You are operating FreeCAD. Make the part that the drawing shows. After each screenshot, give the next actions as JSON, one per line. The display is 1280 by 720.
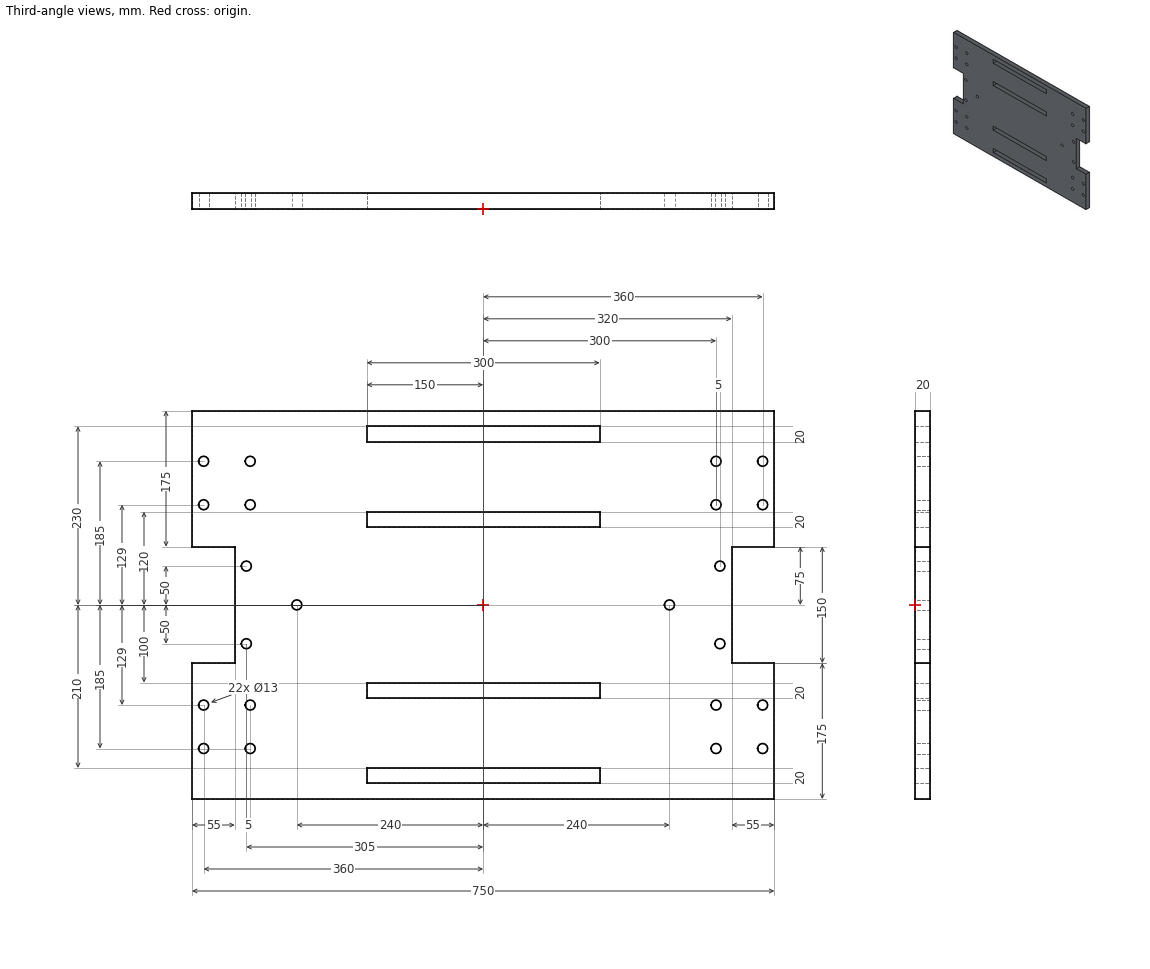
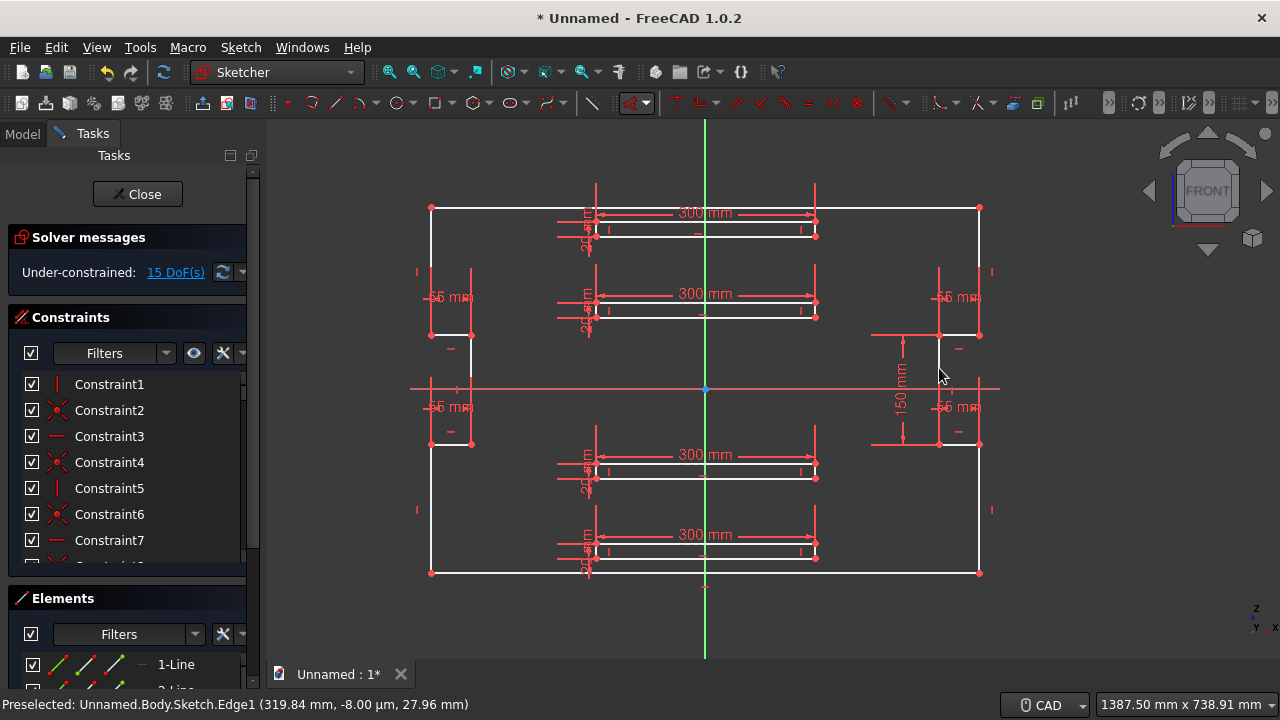
{"action": "left_click", "coordinate": [979, 483]}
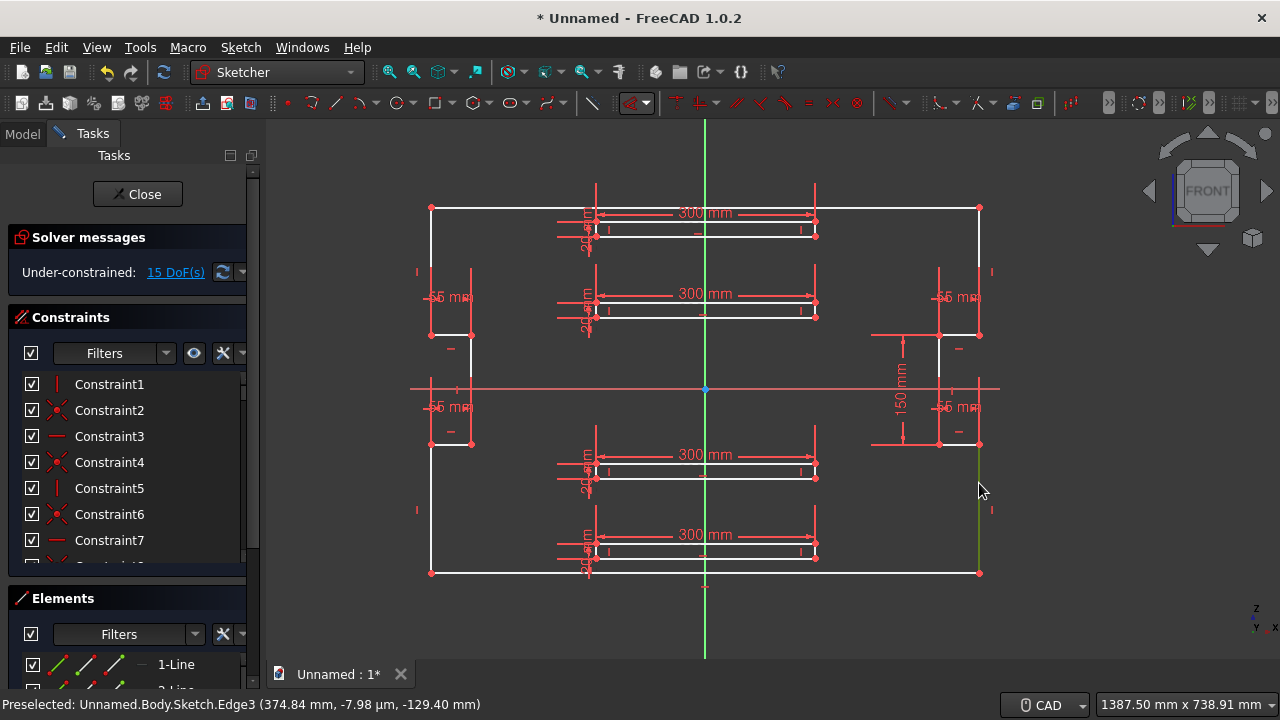
{"action": "left_click", "coordinate": [648, 104]}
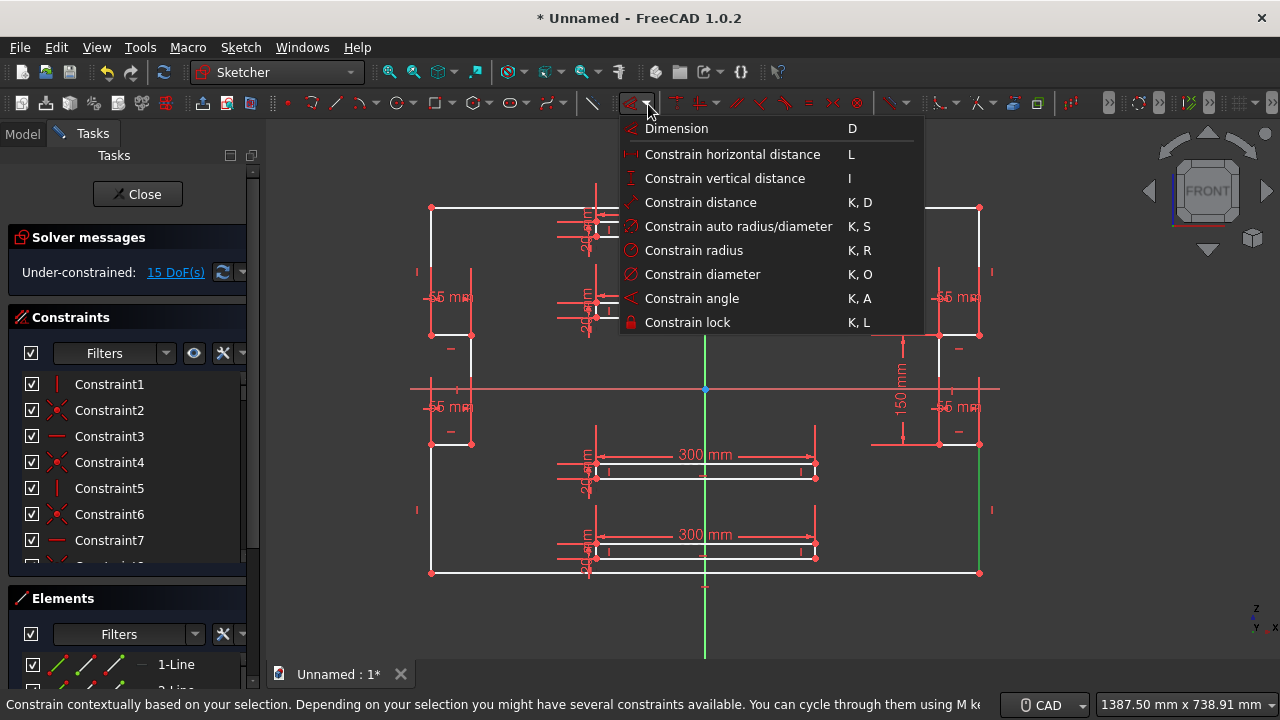
{"action": "left_click", "coordinate": [772, 178]}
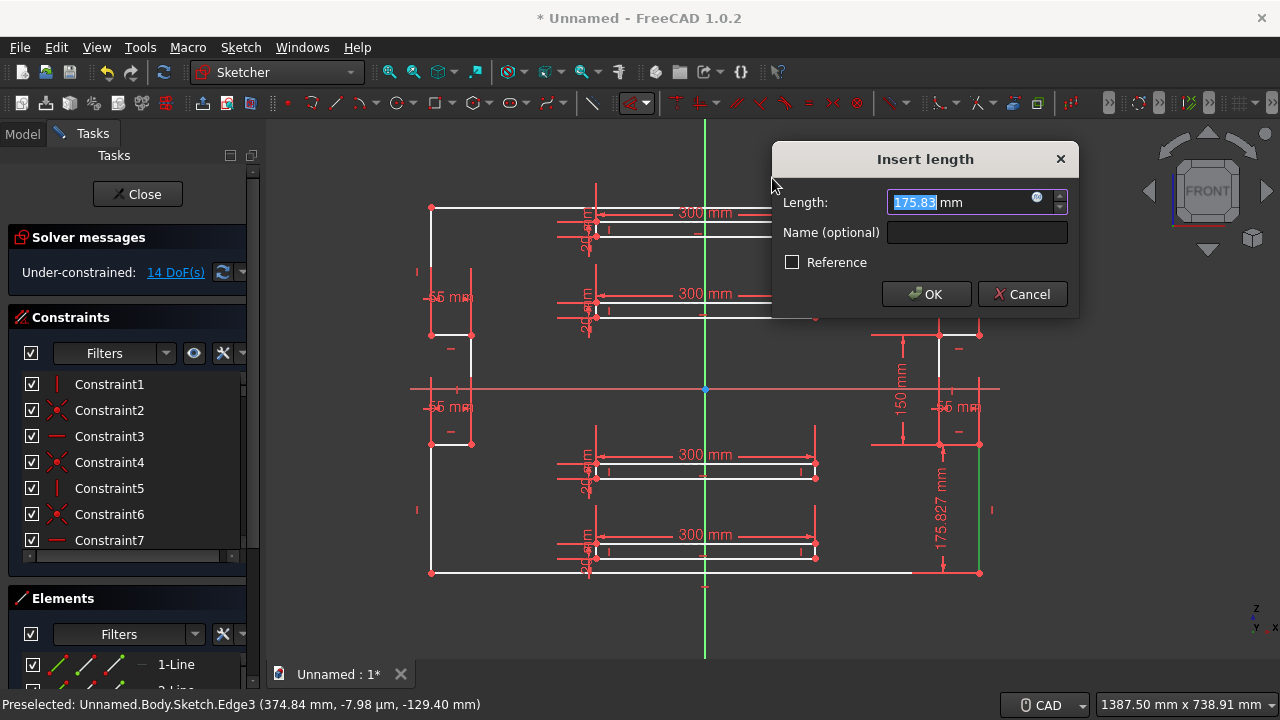
{"action": "type", "text": "175"}
{"action": "key", "text": "Return"}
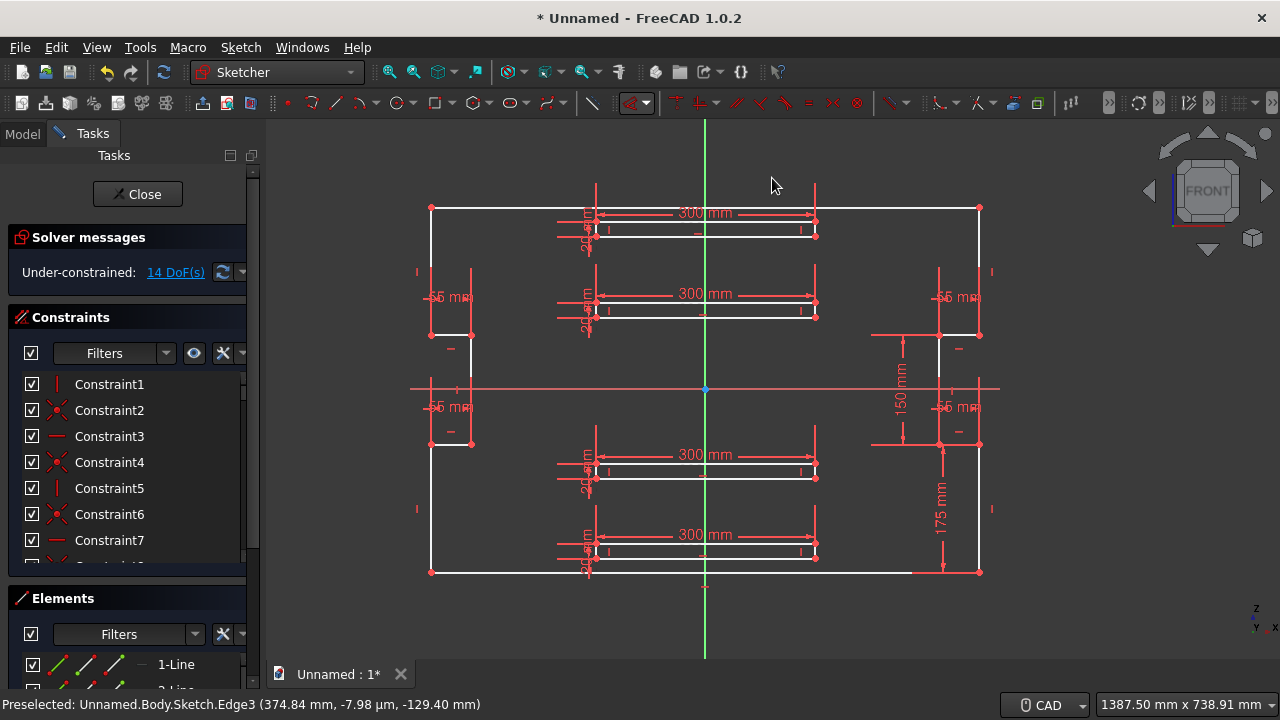
{"action": "left_click", "coordinate": [815, 573]}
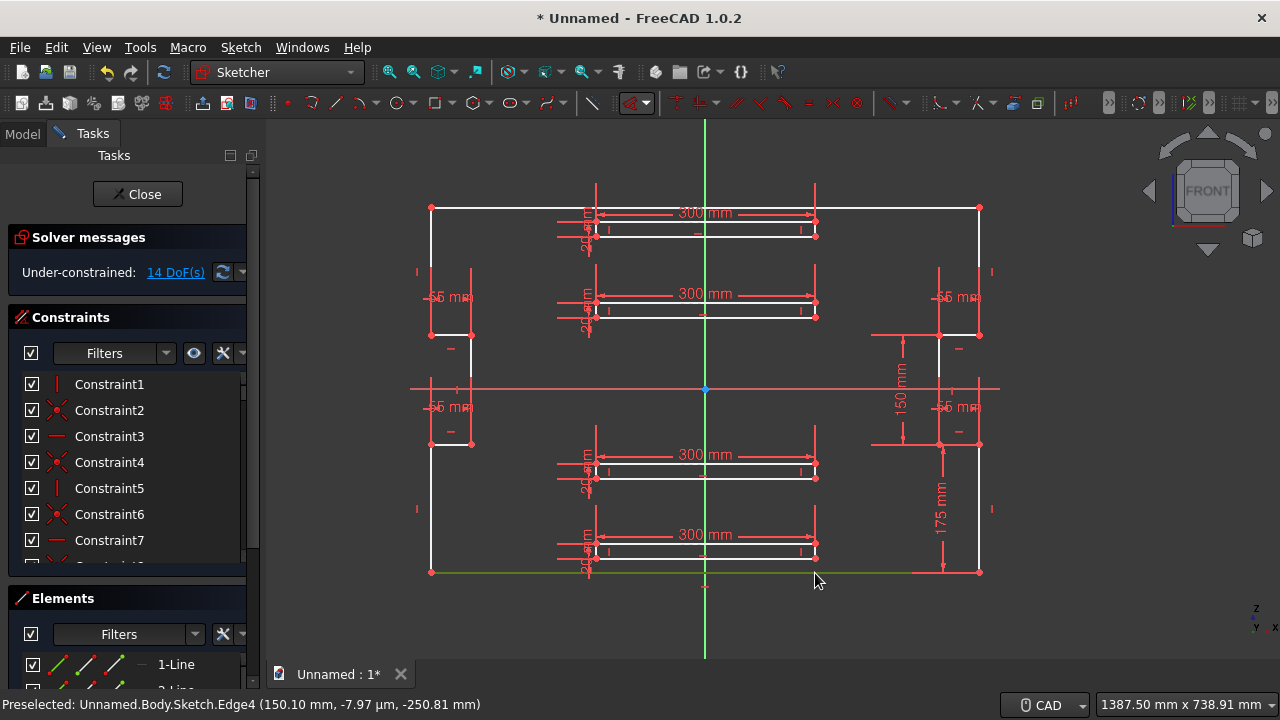
{"action": "left_click", "coordinate": [648, 104]}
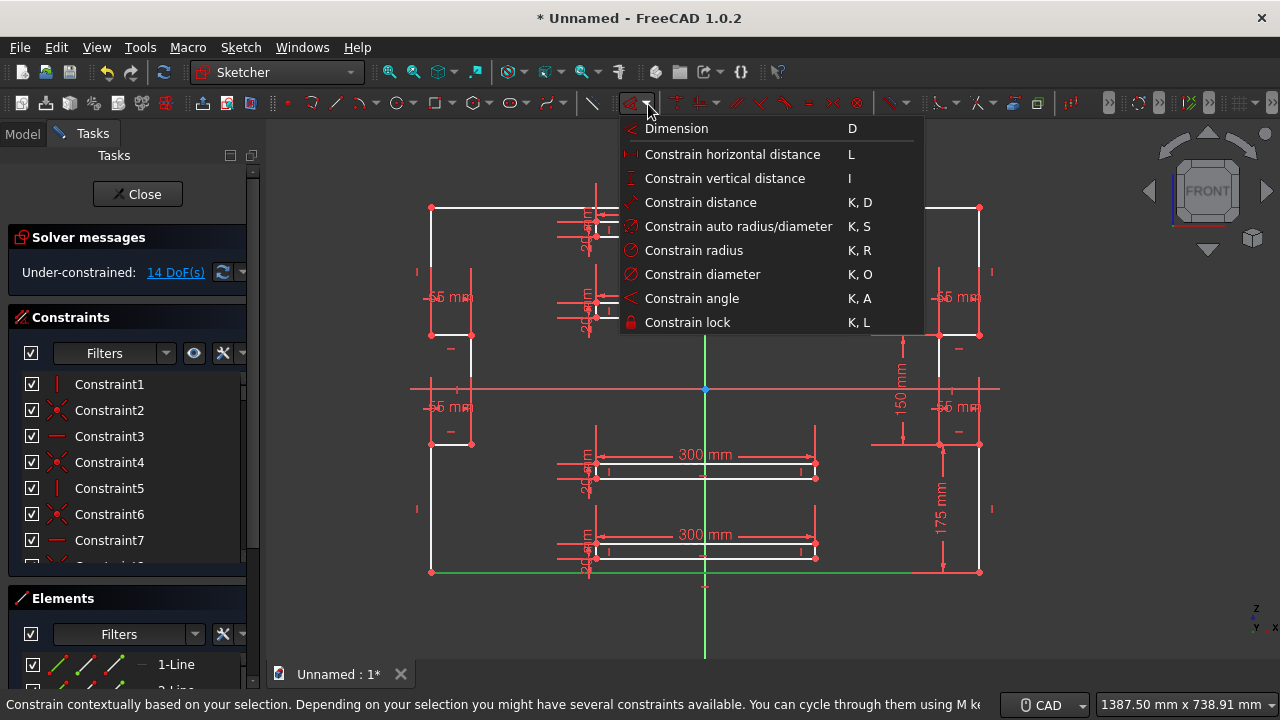
{"action": "left_click", "coordinate": [772, 154]}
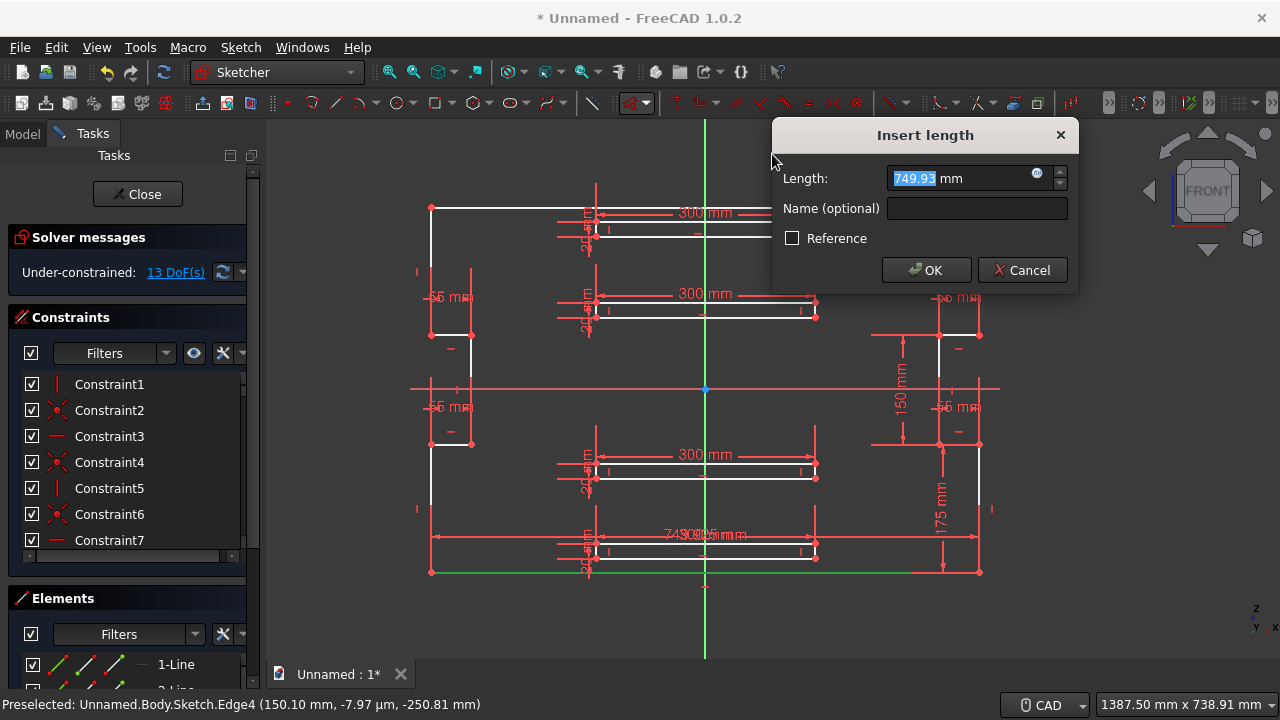
{"action": "type", "text": "750"}
{"action": "key", "text": "Return"}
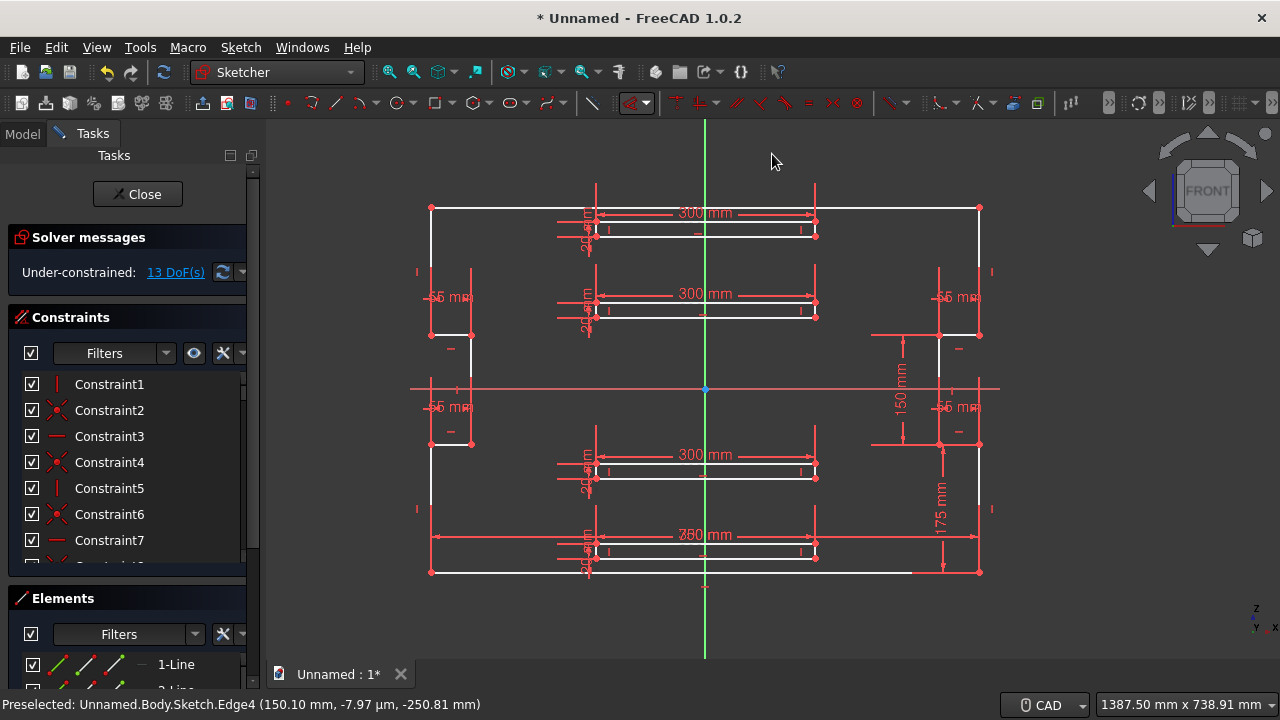
{"action": "left_click", "coordinate": [431, 534]}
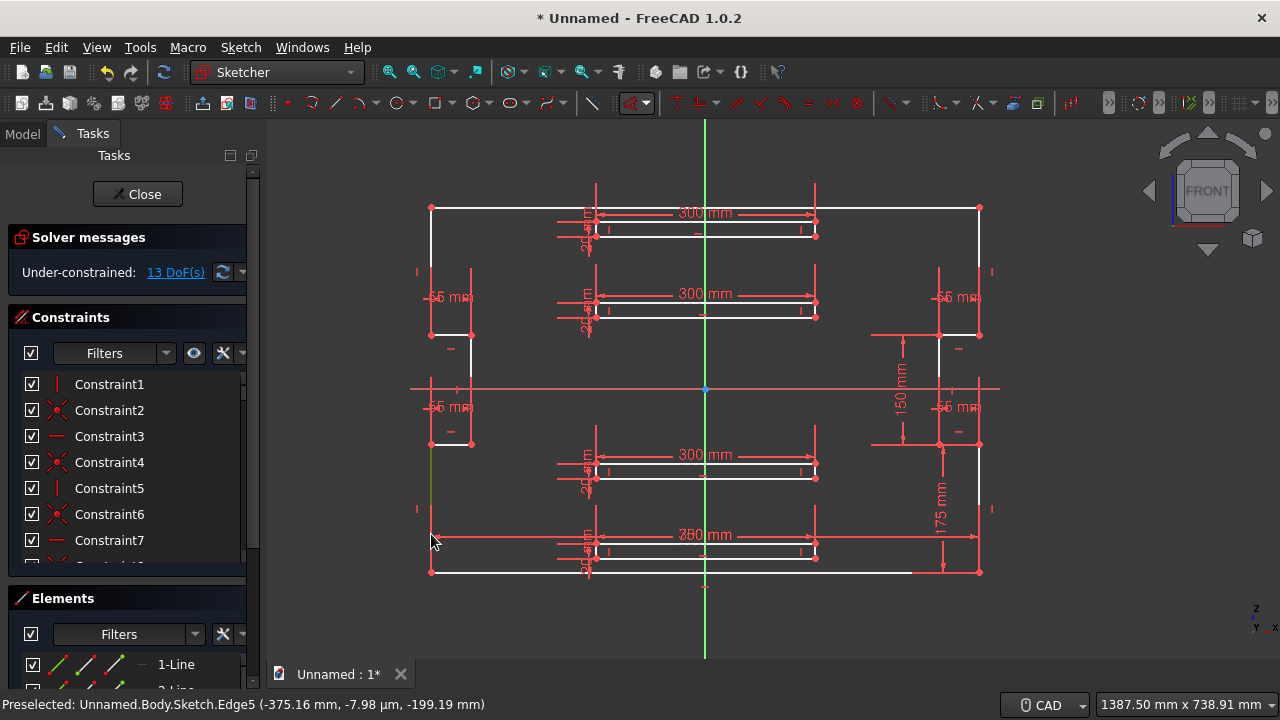
{"action": "key", "text": "i"}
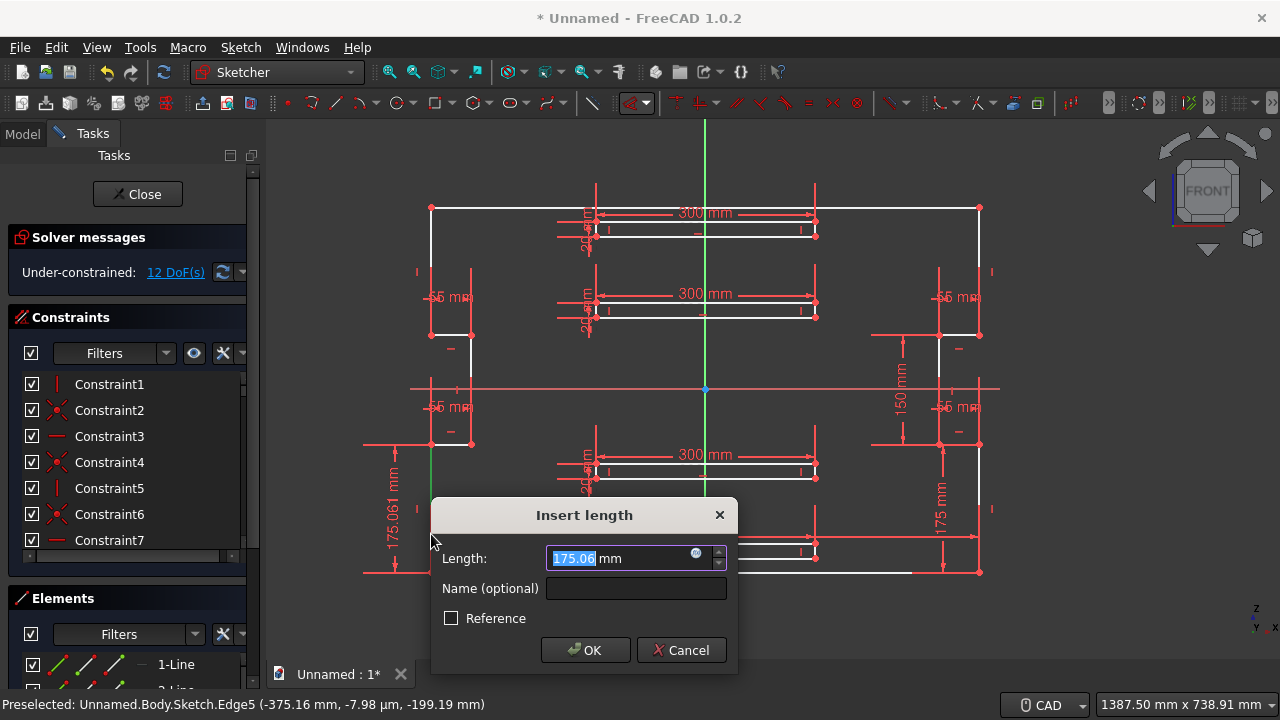
{"action": "type", "text": "175"}
{"action": "key", "text": "Return"}